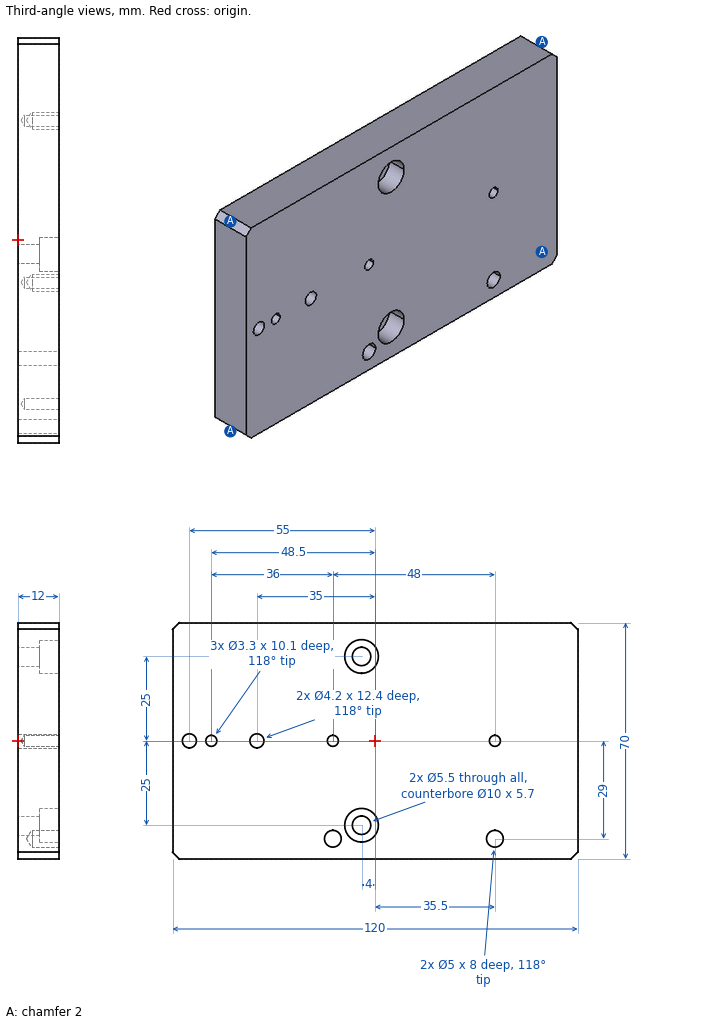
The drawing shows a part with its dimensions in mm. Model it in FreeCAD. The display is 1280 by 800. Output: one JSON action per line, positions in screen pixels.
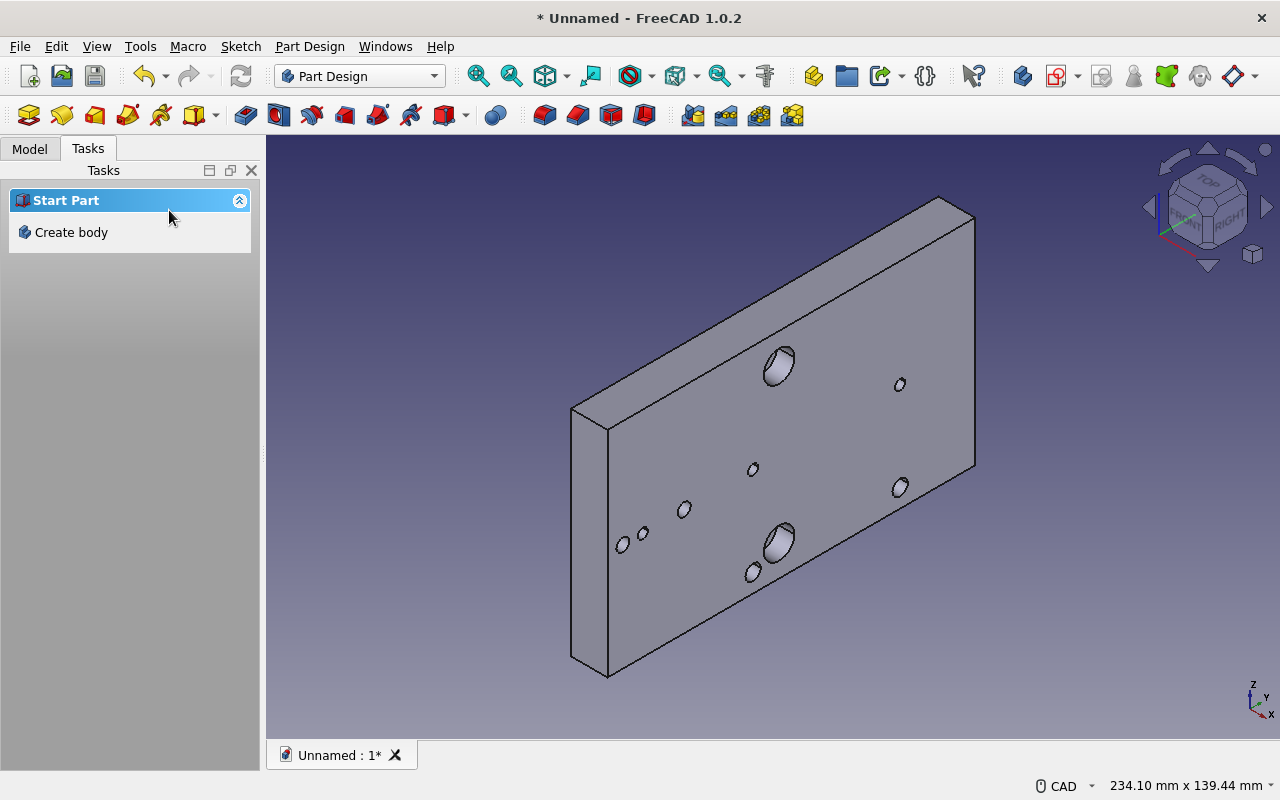
{"action": "left_click", "coordinate": [589, 418]}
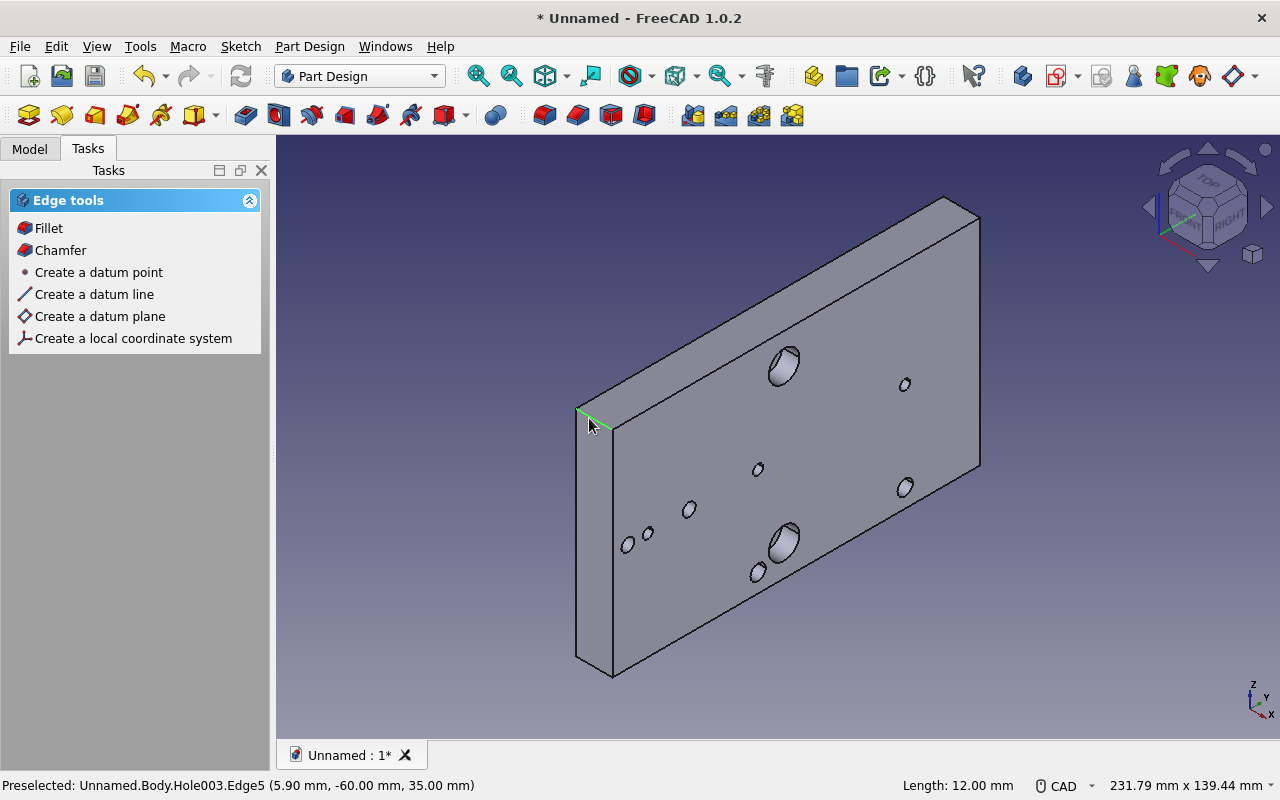
{"action": "key", "text": "2"}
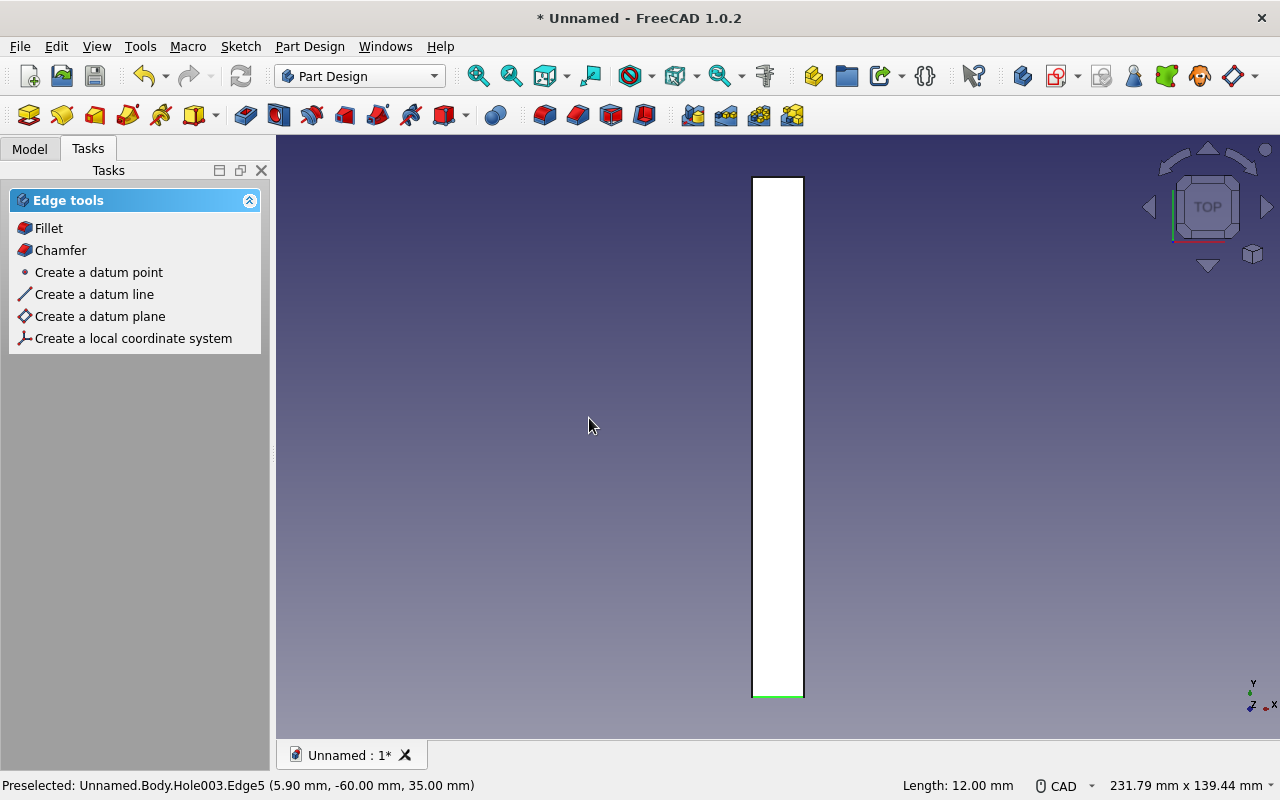
{"action": "left_click", "coordinate": [778, 176], "text": "ctrl"}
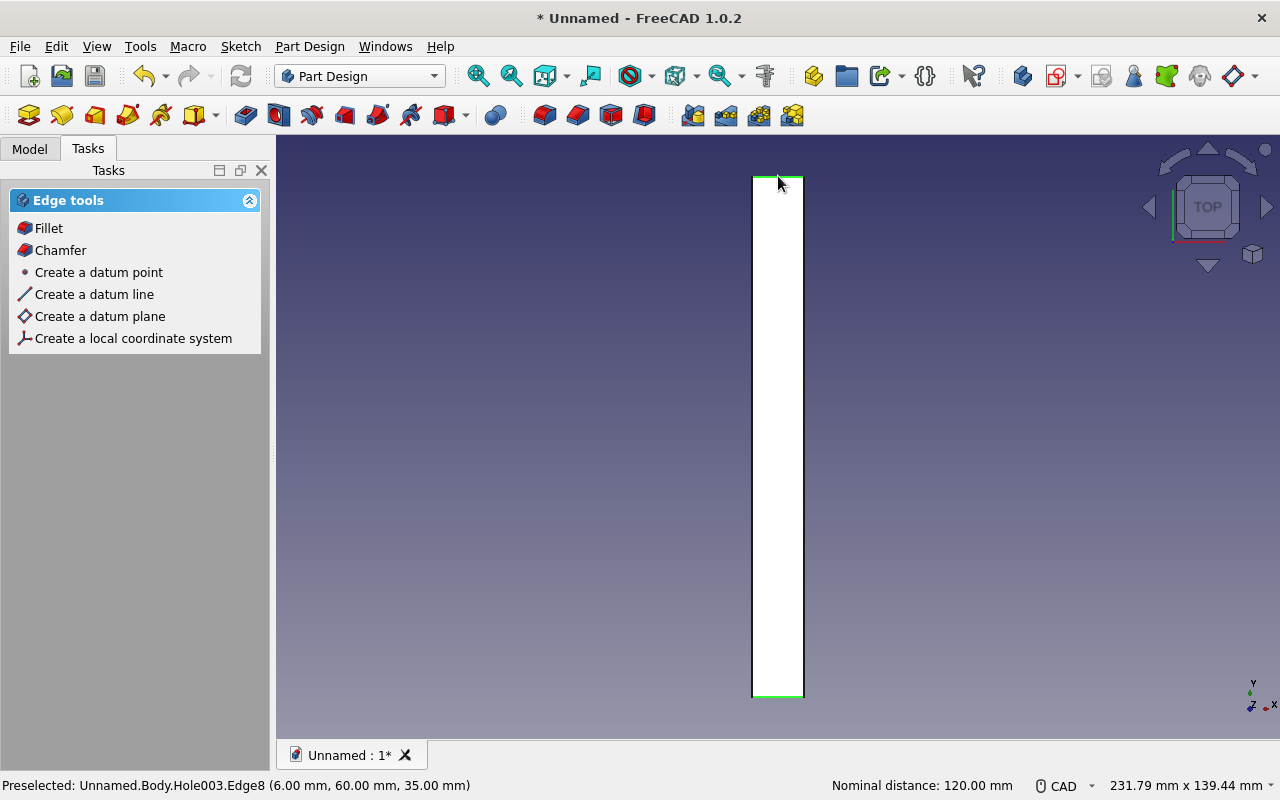
{"action": "key", "text": "0"}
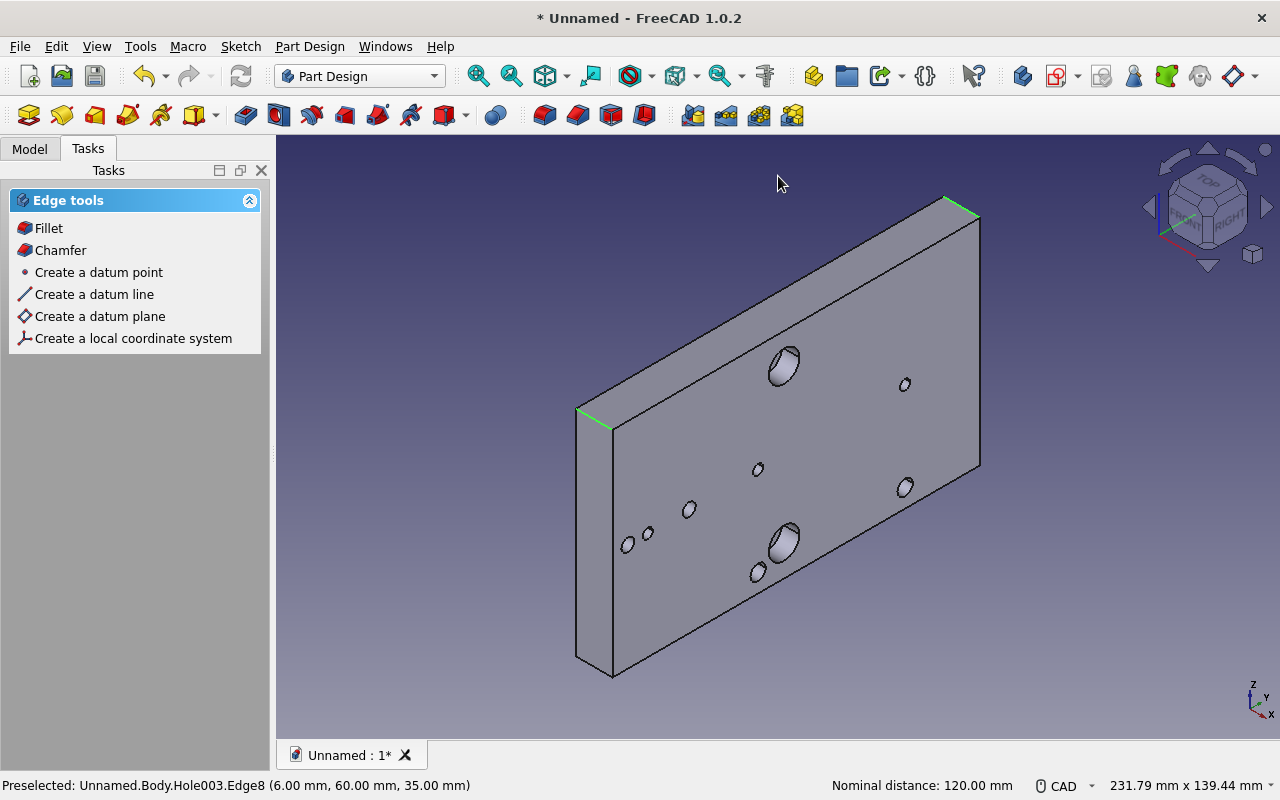
{"action": "key", "text": "1"}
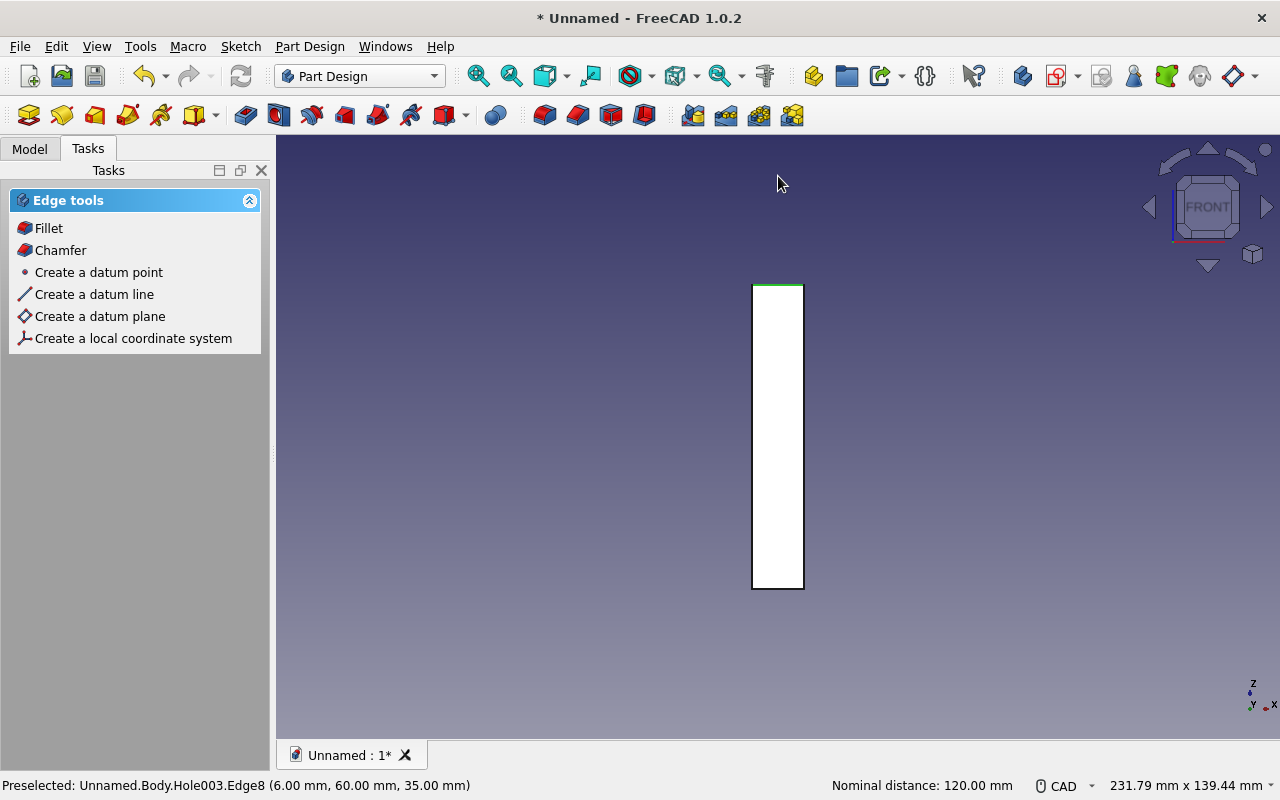
{"action": "left_click", "coordinate": [778, 588], "text": "ctrl"}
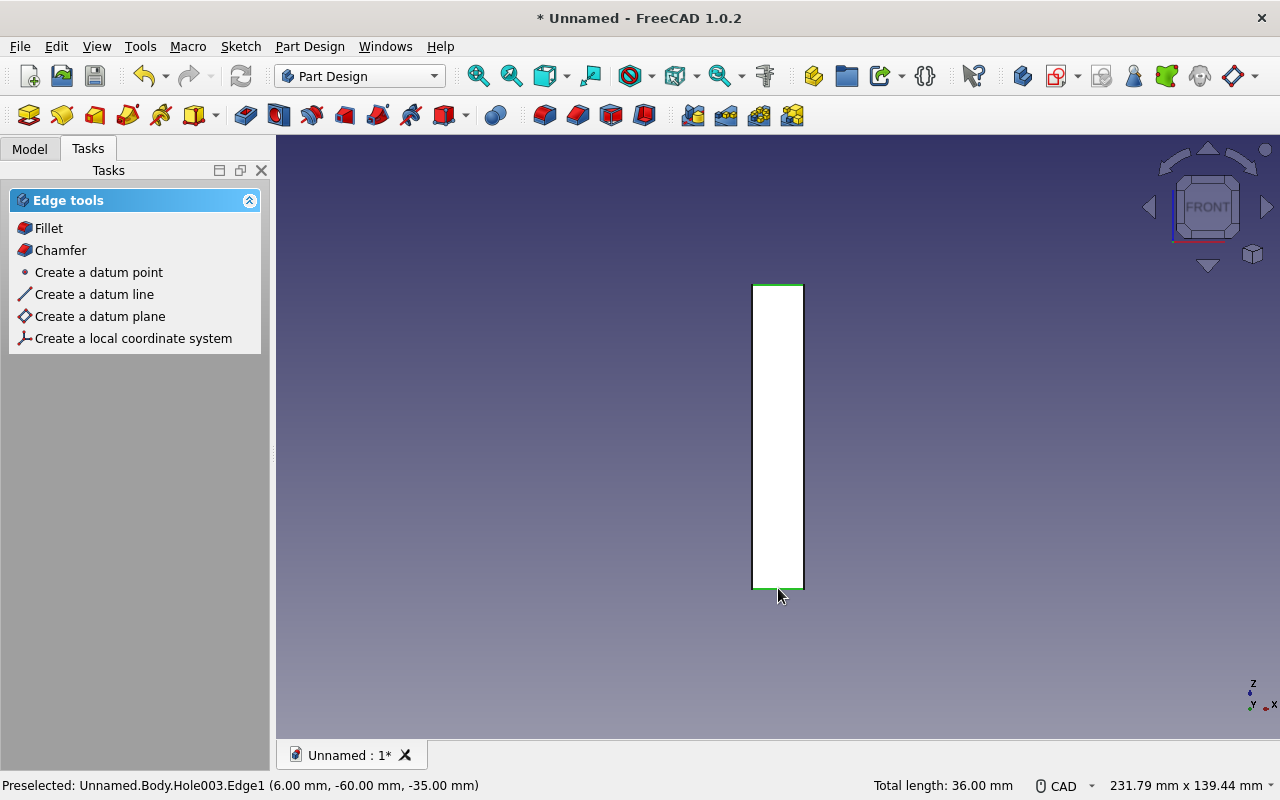
{"action": "key", "text": "3"}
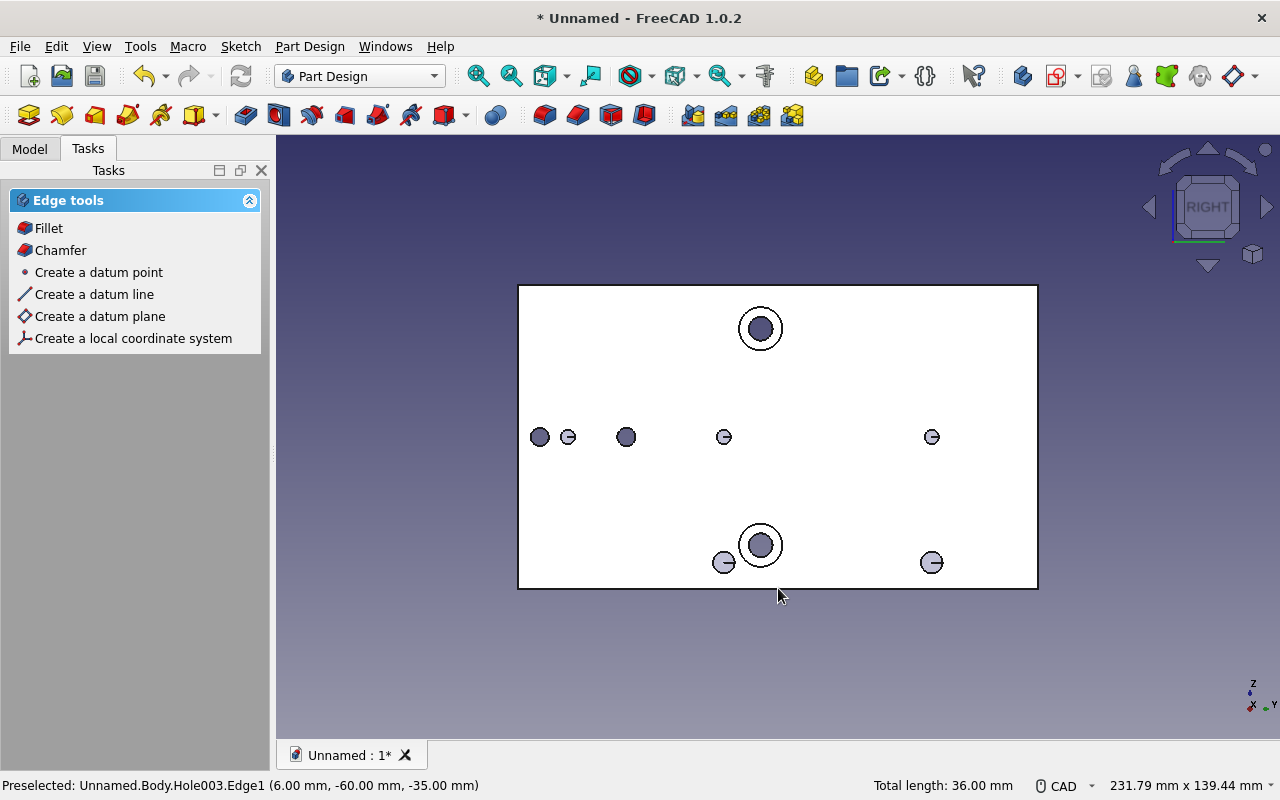
{"action": "key", "text": "5"}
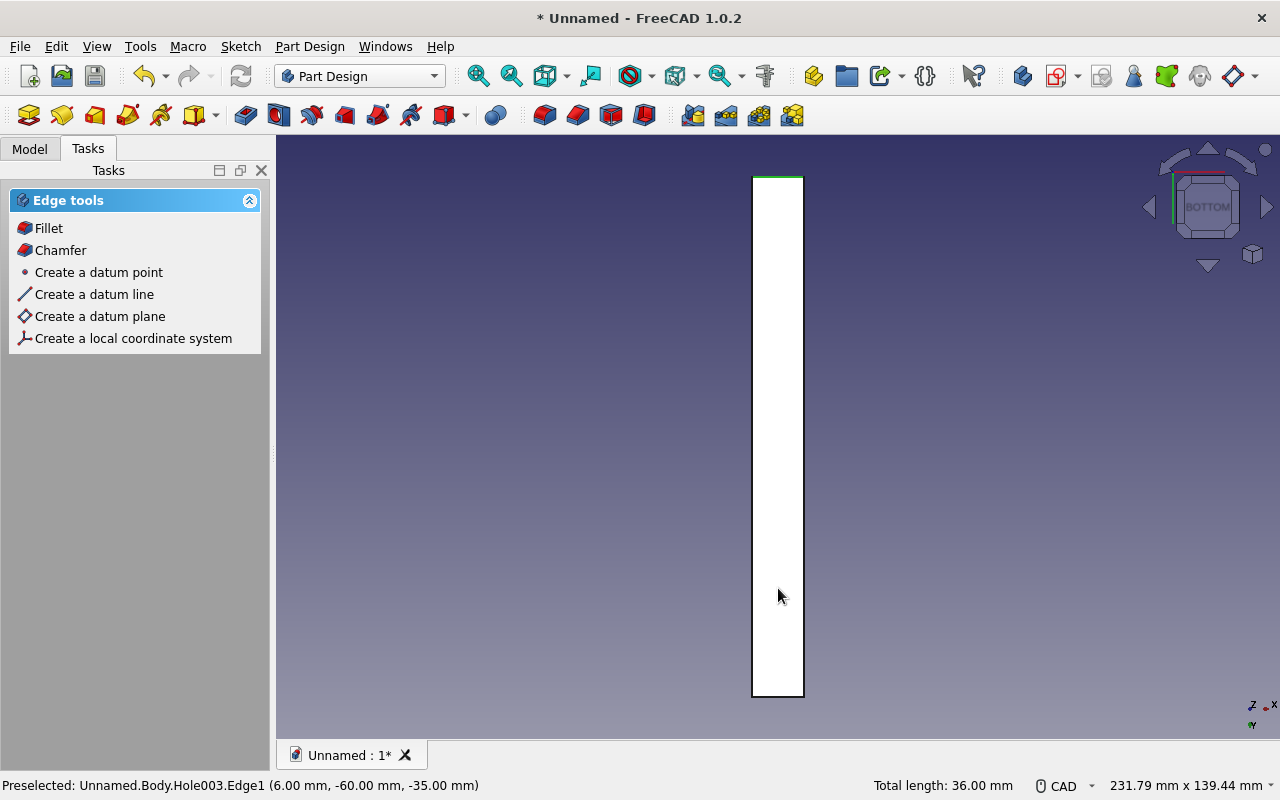
{"action": "left_click", "coordinate": [778, 696], "text": "ctrl"}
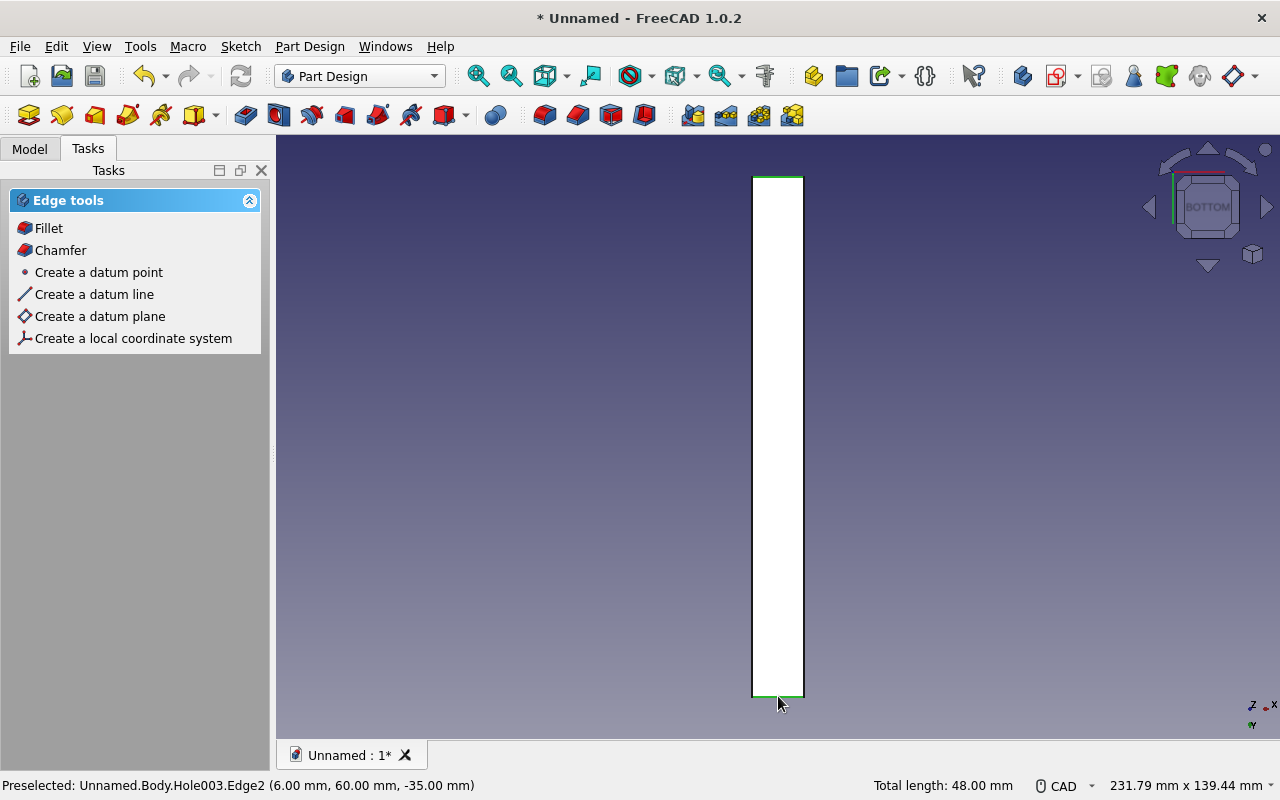
{"action": "left_click", "coordinate": [578, 116]}